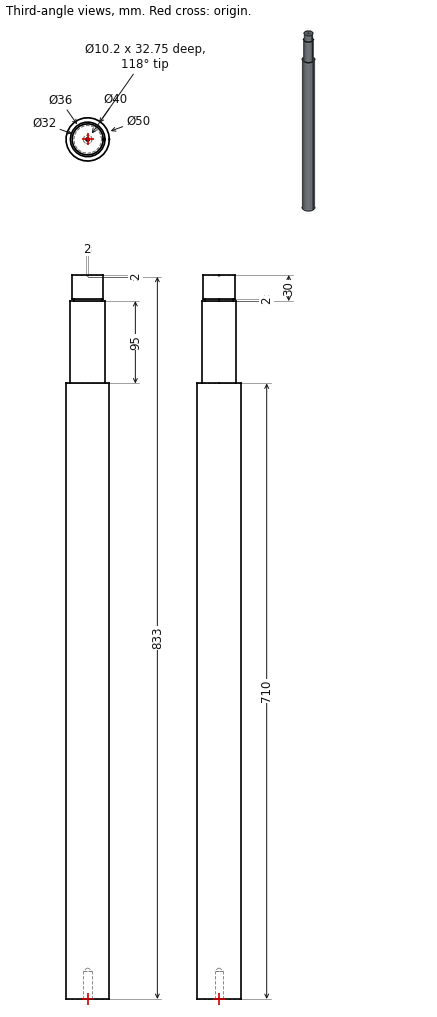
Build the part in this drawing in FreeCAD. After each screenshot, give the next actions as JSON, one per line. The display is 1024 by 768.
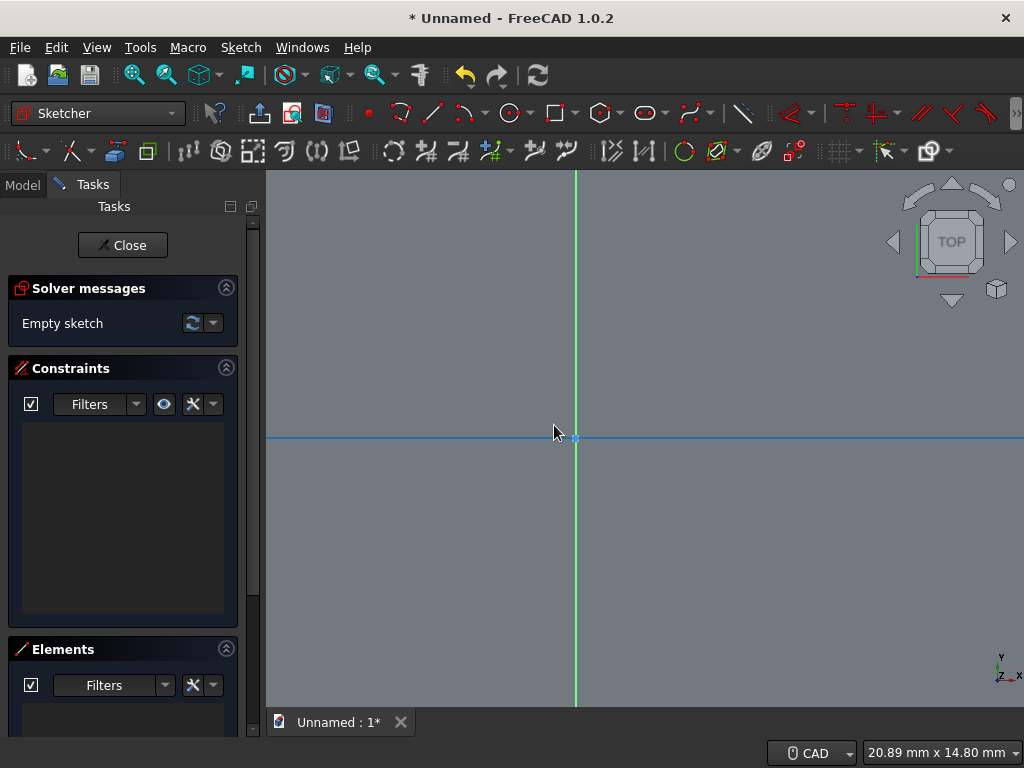
{"action": "left_click", "coordinate": [510, 114]}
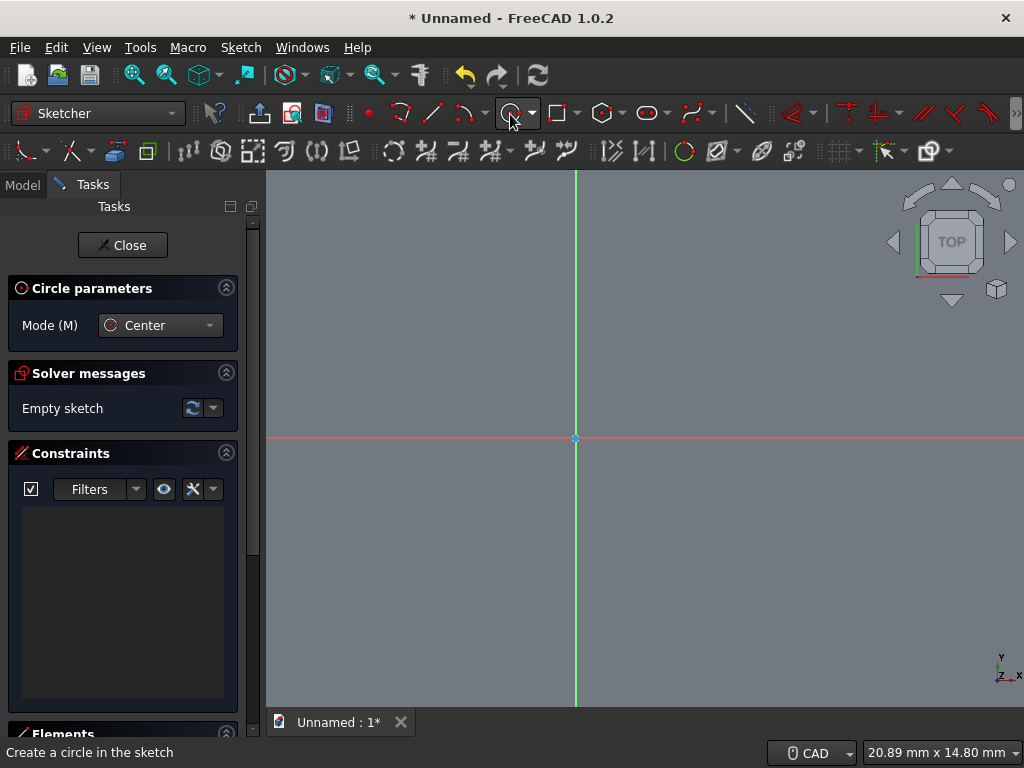
{"action": "left_click", "coordinate": [576, 438]}
{"action": "mouse_move", "coordinate": [707, 307]}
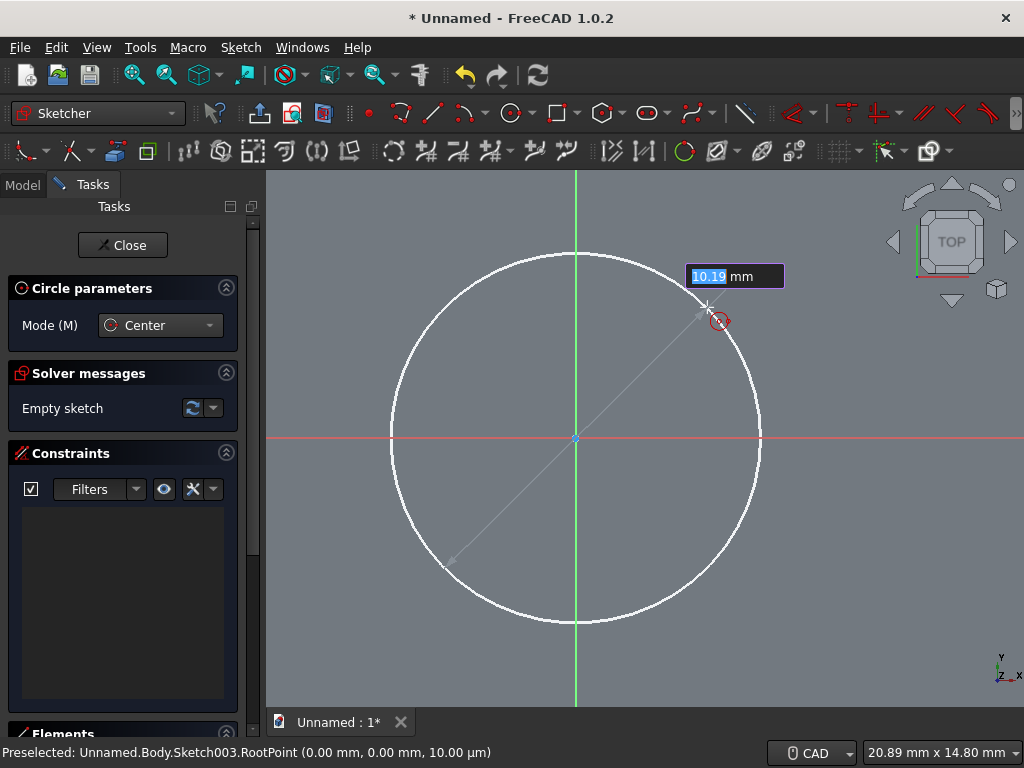
{"action": "type", "text": "10.2"}
{"action": "key", "text": "Return"}
{"action": "key", "text": "Escape"}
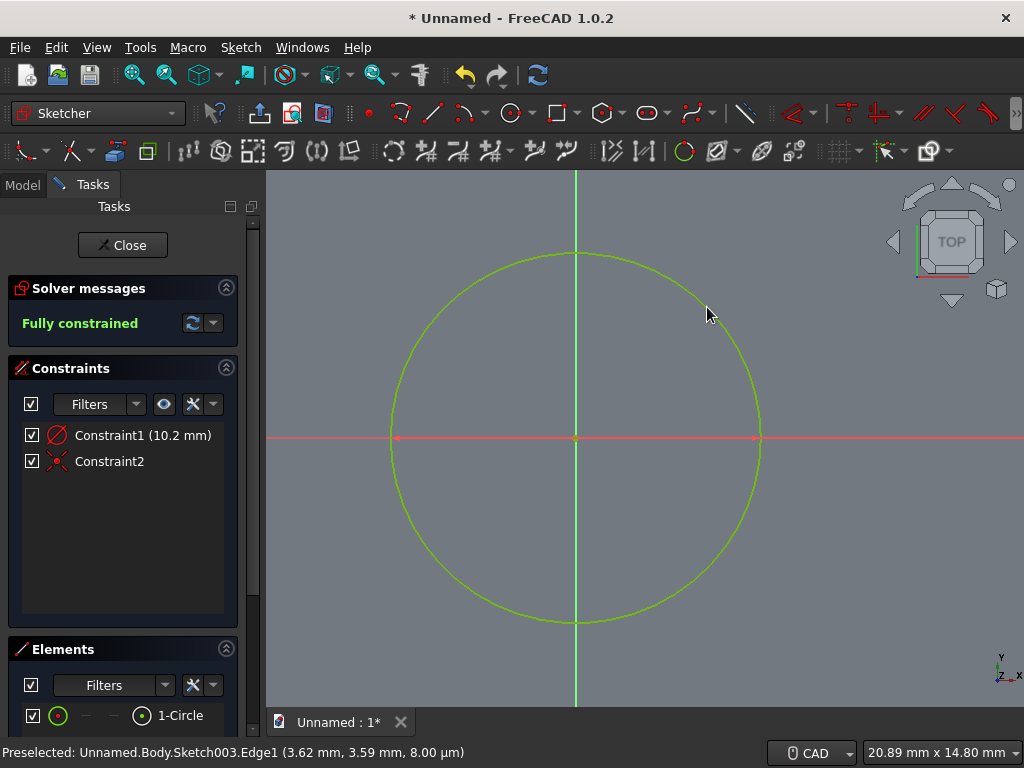
{"action": "left_click", "coordinate": [123, 245]}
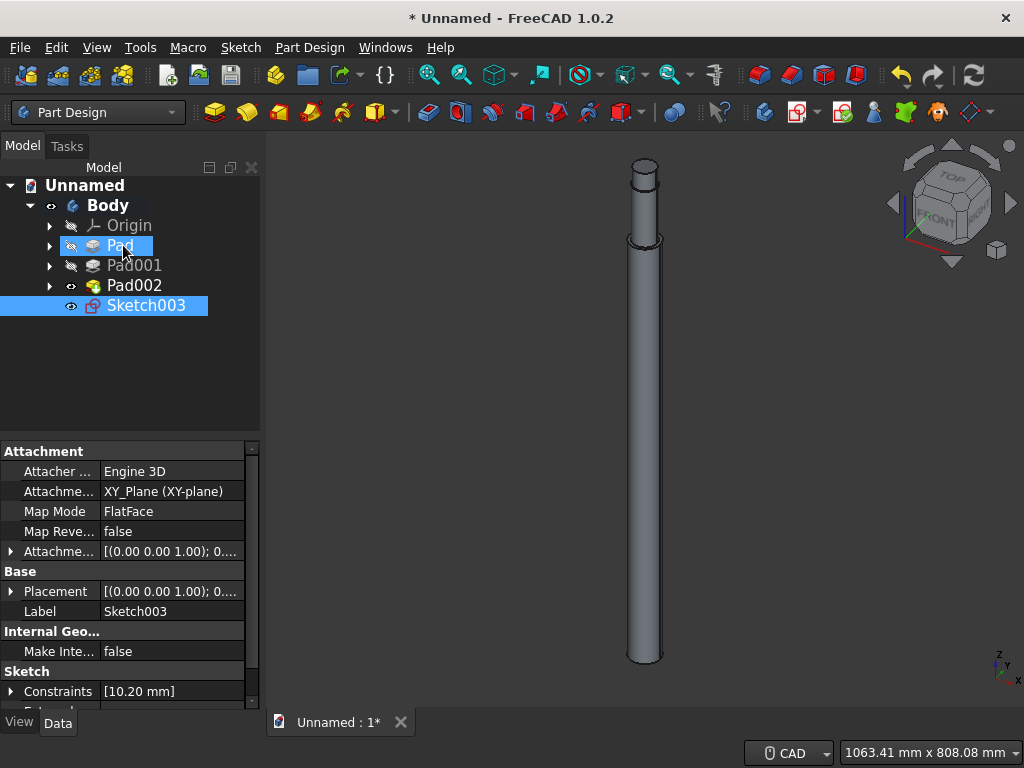
{"action": "left_click", "coordinate": [462, 112]}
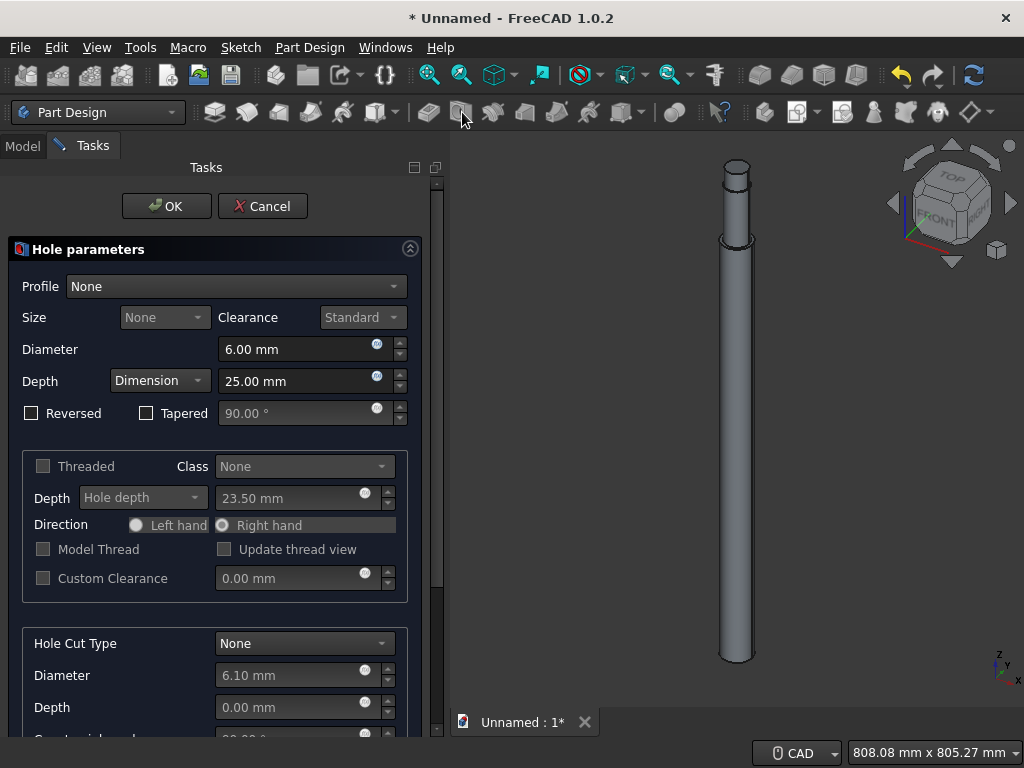
{"action": "triple_click", "coordinate": [305, 349]}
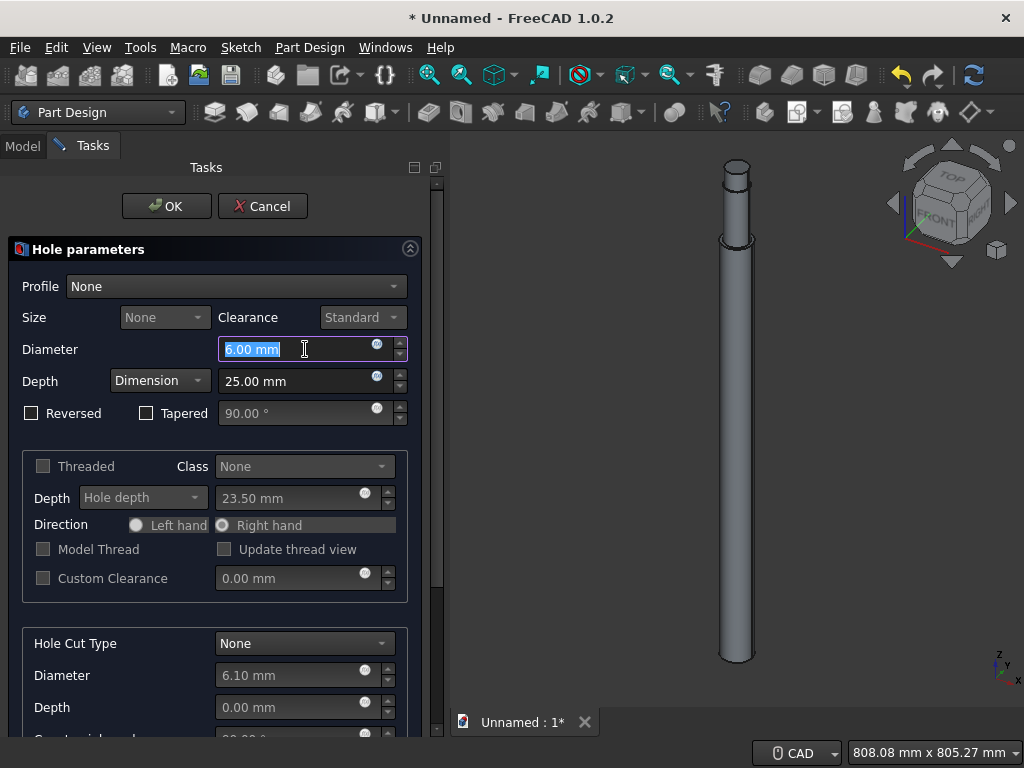
{"action": "type", "text": "10.2"}
{"action": "key", "text": "Tab"}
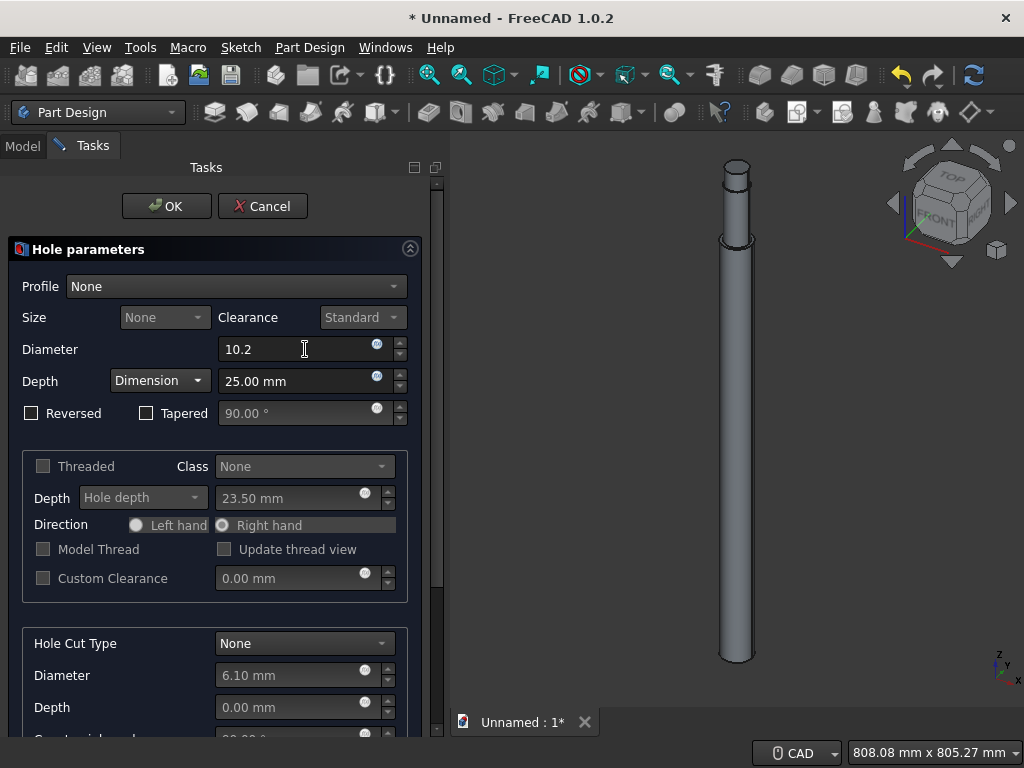
{"action": "triple_click", "coordinate": [305, 381]}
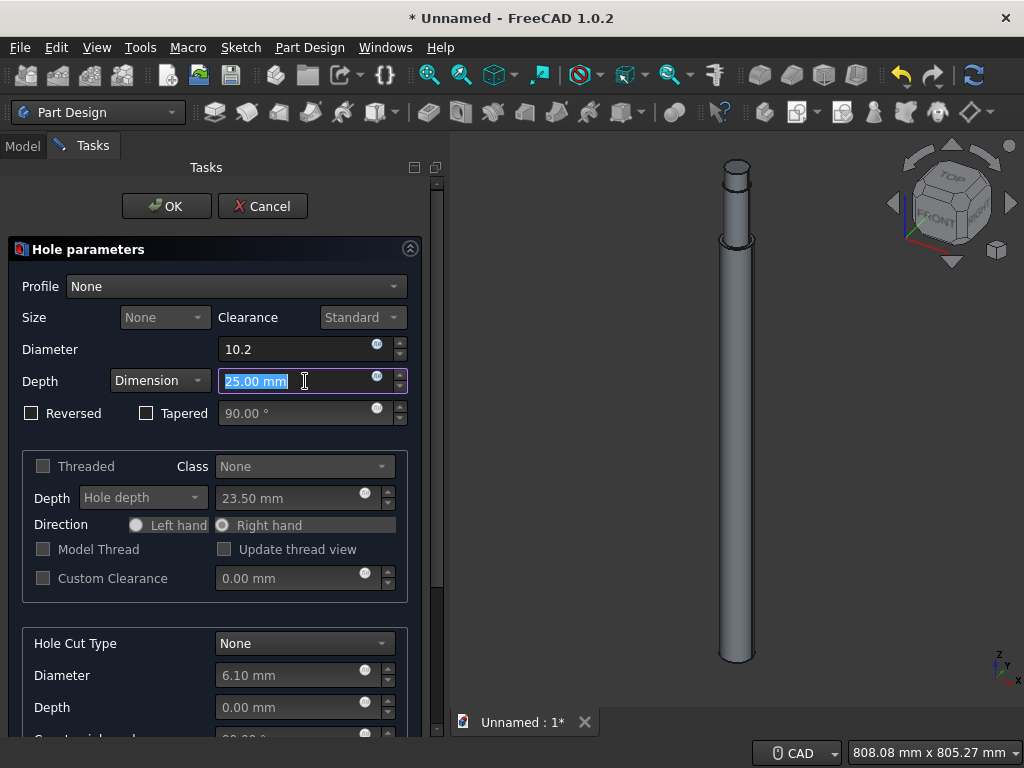
{"action": "type", "text": "32.75"}
{"action": "key", "text": "Tab"}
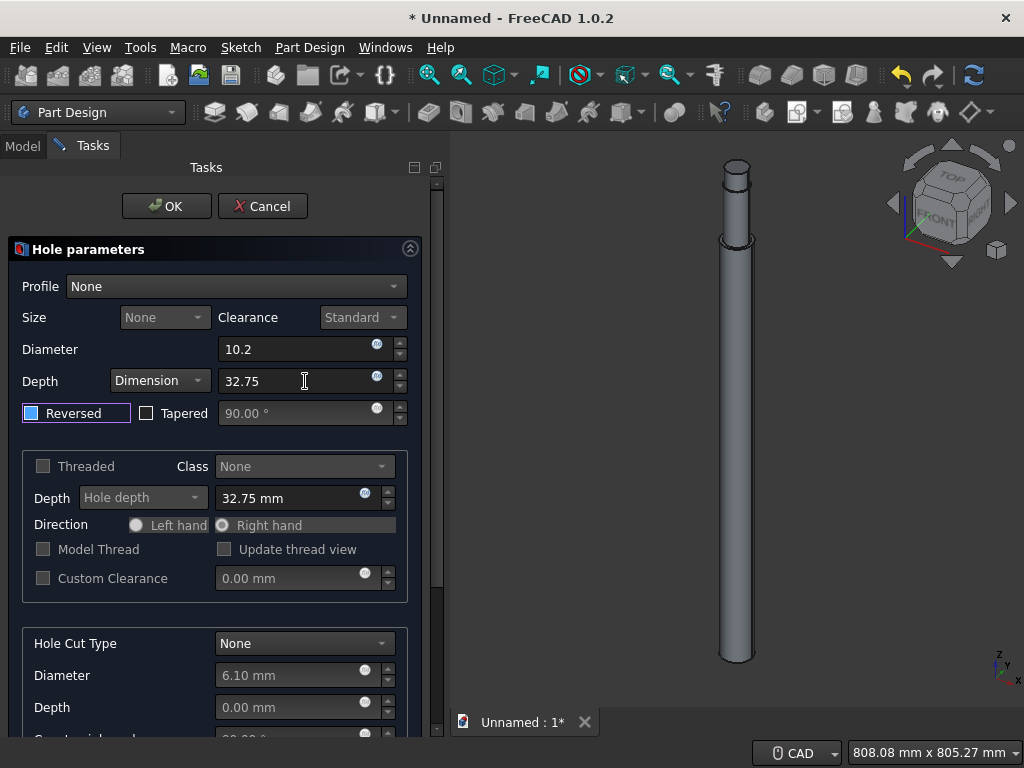
{"action": "left_click", "coordinate": [30, 413]}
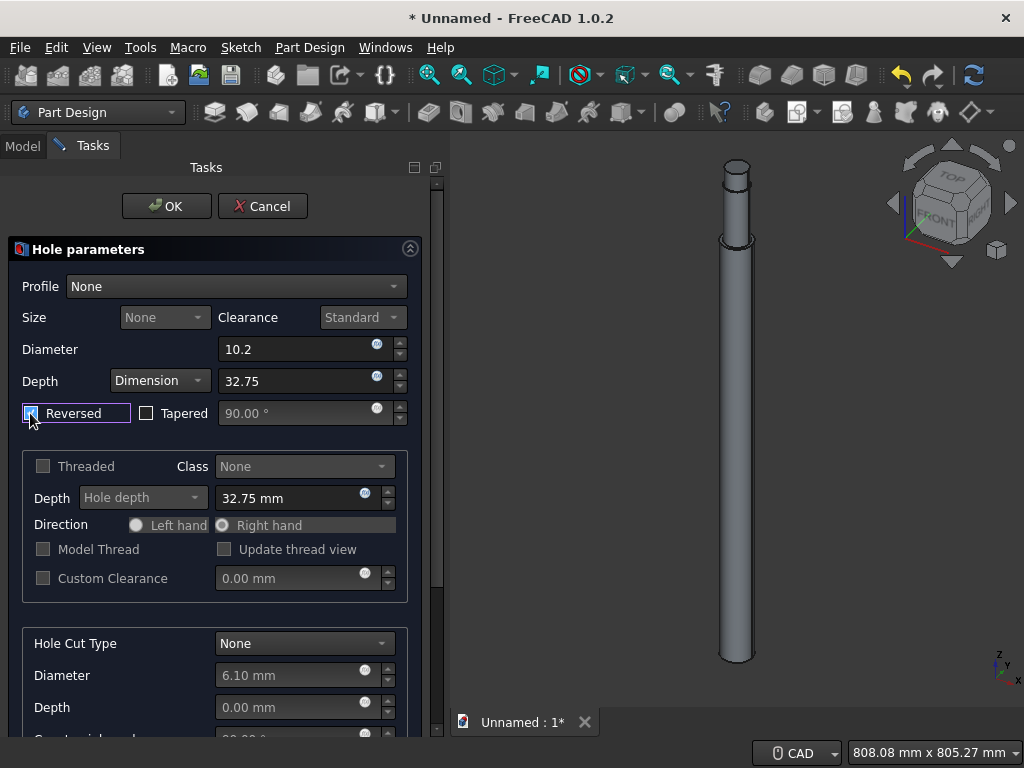
{"action": "left_click", "coordinate": [167, 206]}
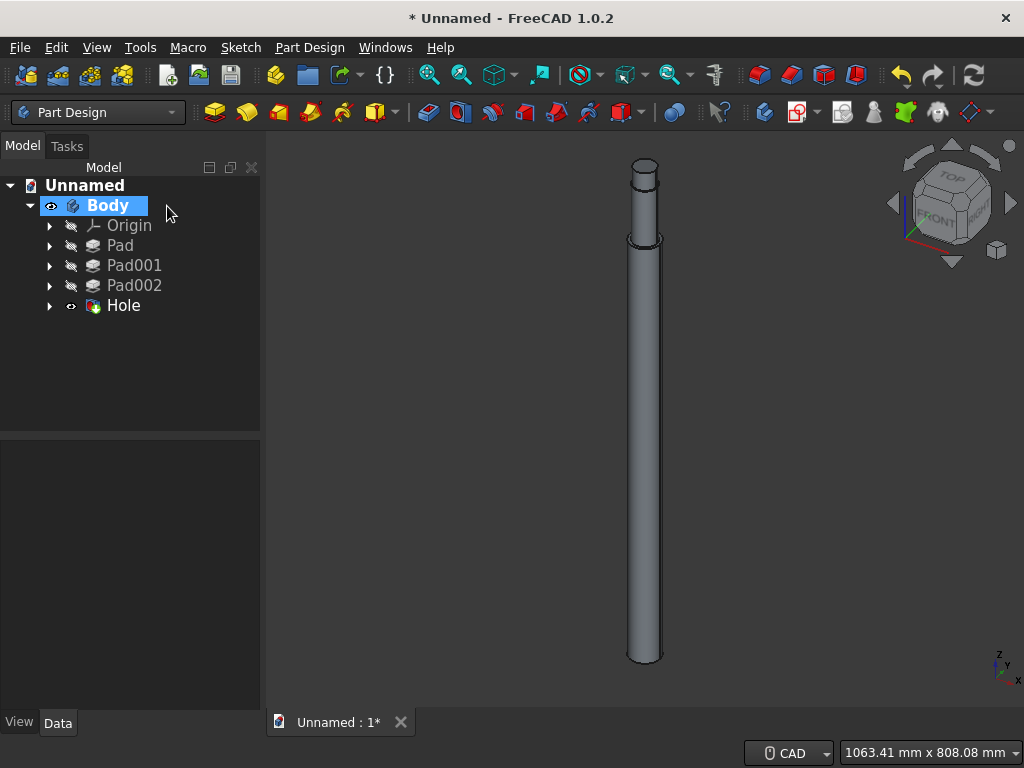
{"action": "left_click", "coordinate": [798, 112]}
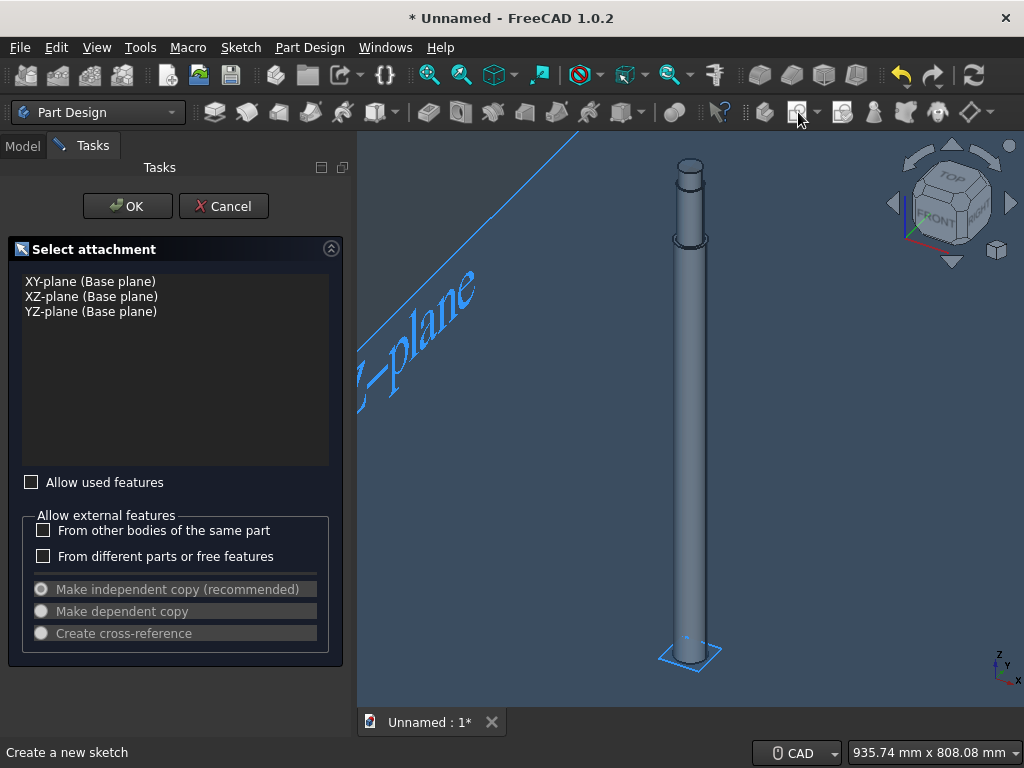
{"action": "left_click", "coordinate": [82, 296]}